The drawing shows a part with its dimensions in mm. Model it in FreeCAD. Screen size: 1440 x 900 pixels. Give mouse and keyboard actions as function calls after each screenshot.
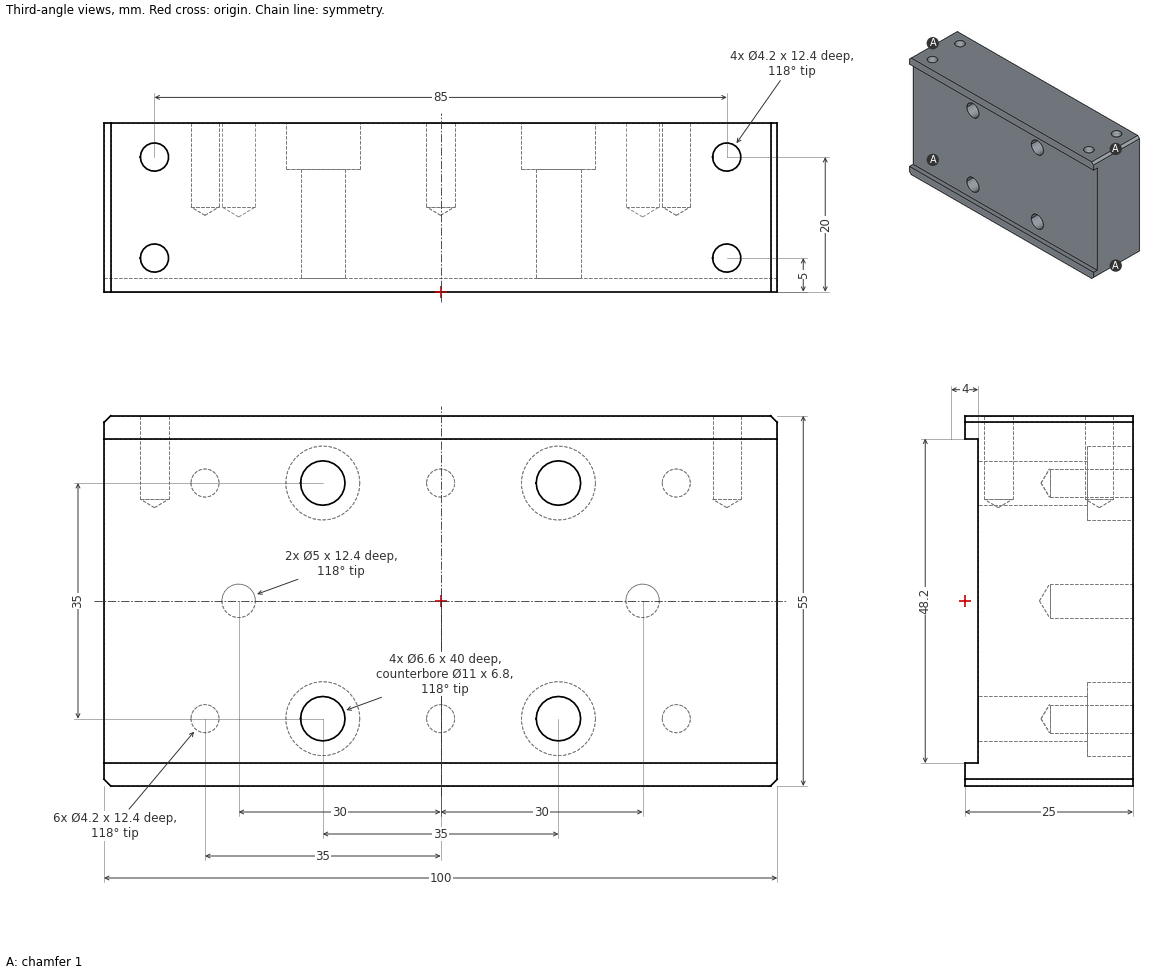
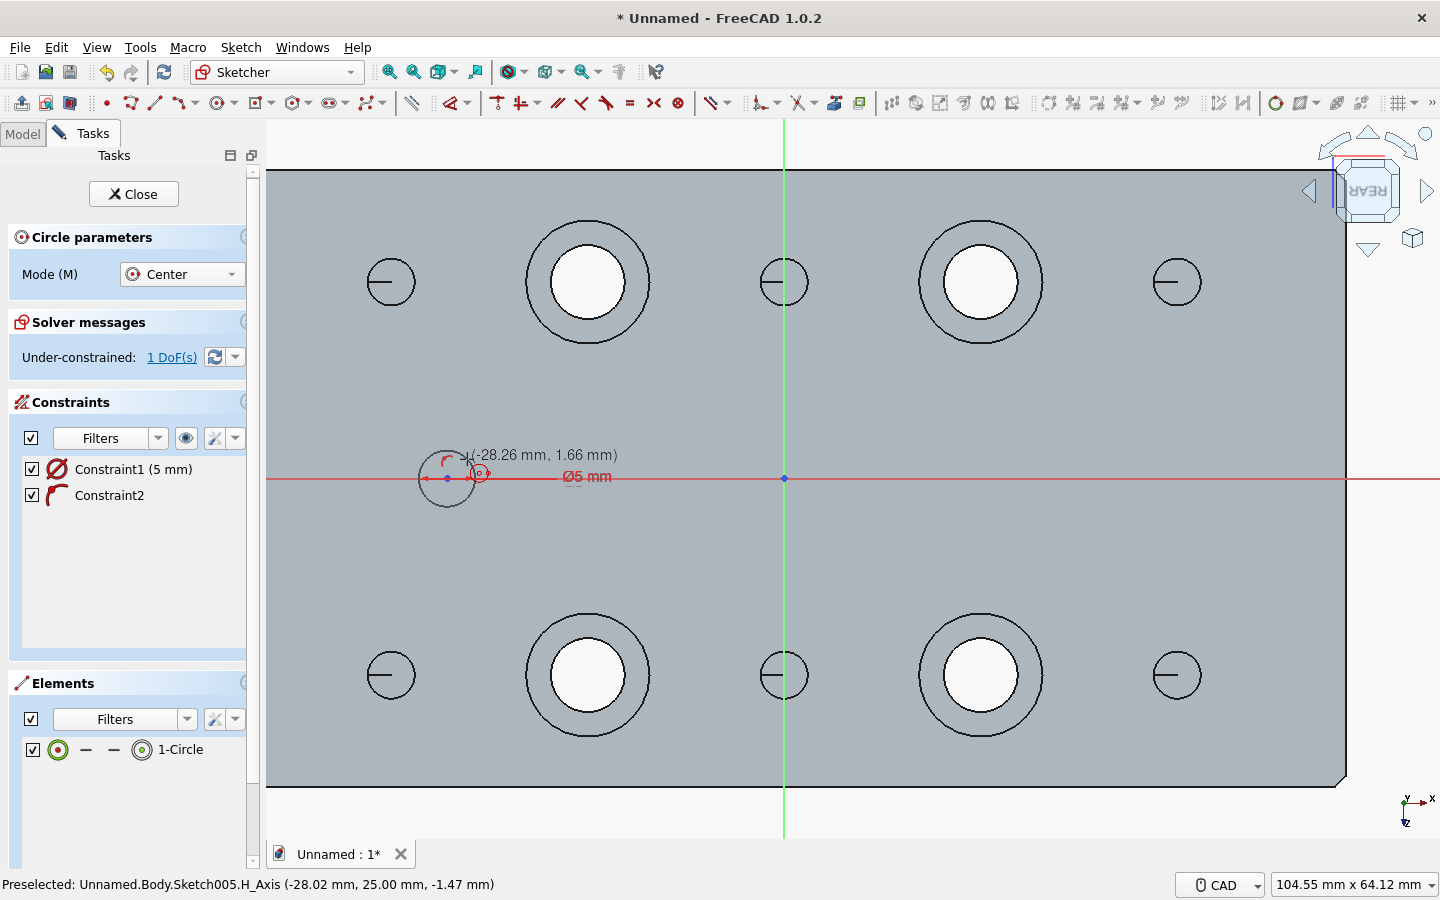
click(1121, 479)
move(1141, 459)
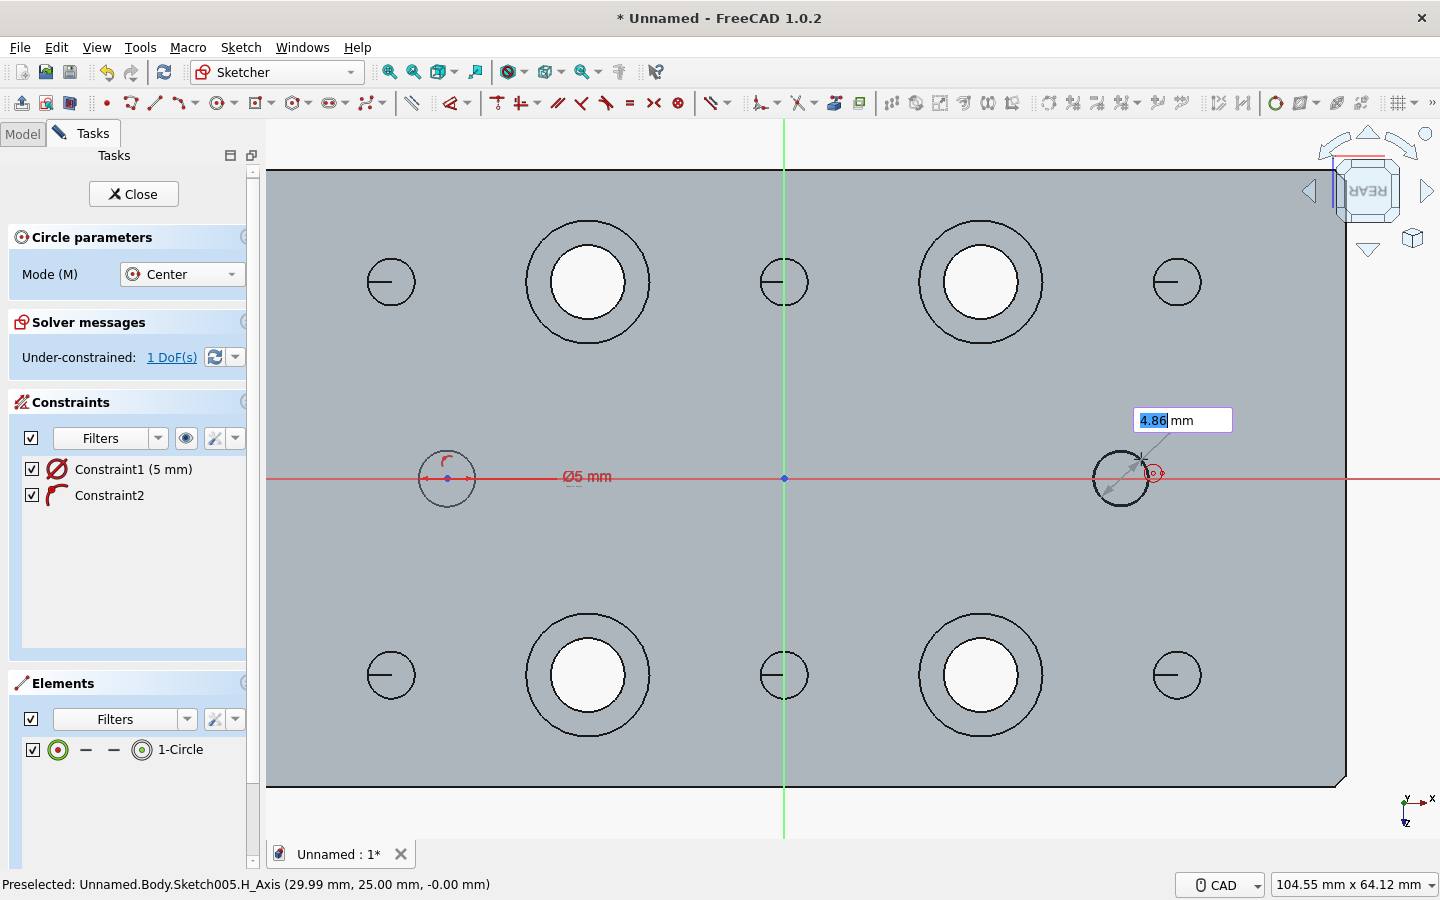
text(5)
key(Return)
key(Escape)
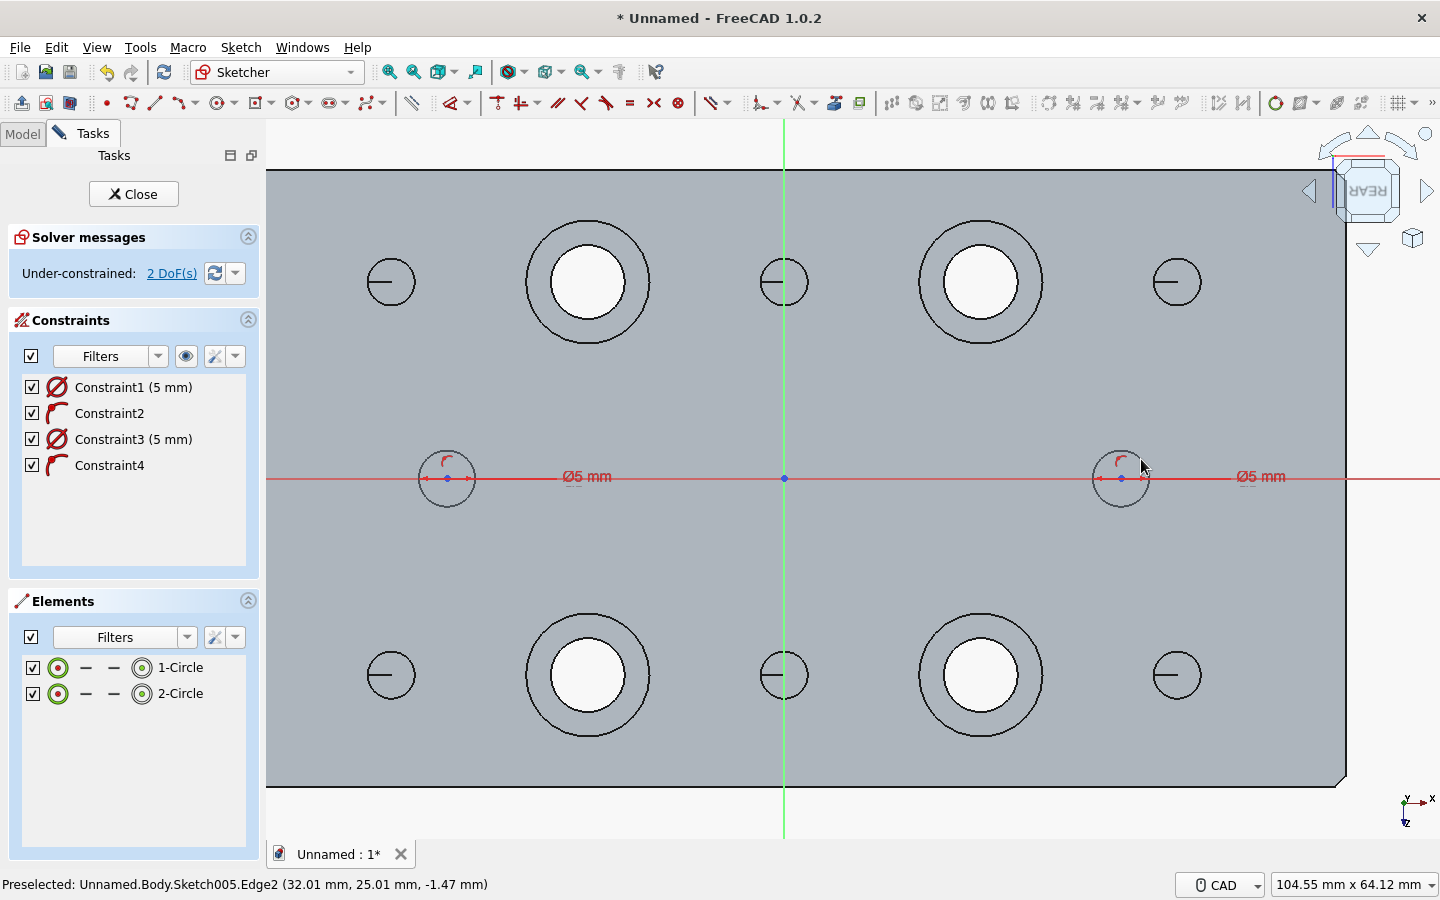
click(450, 104)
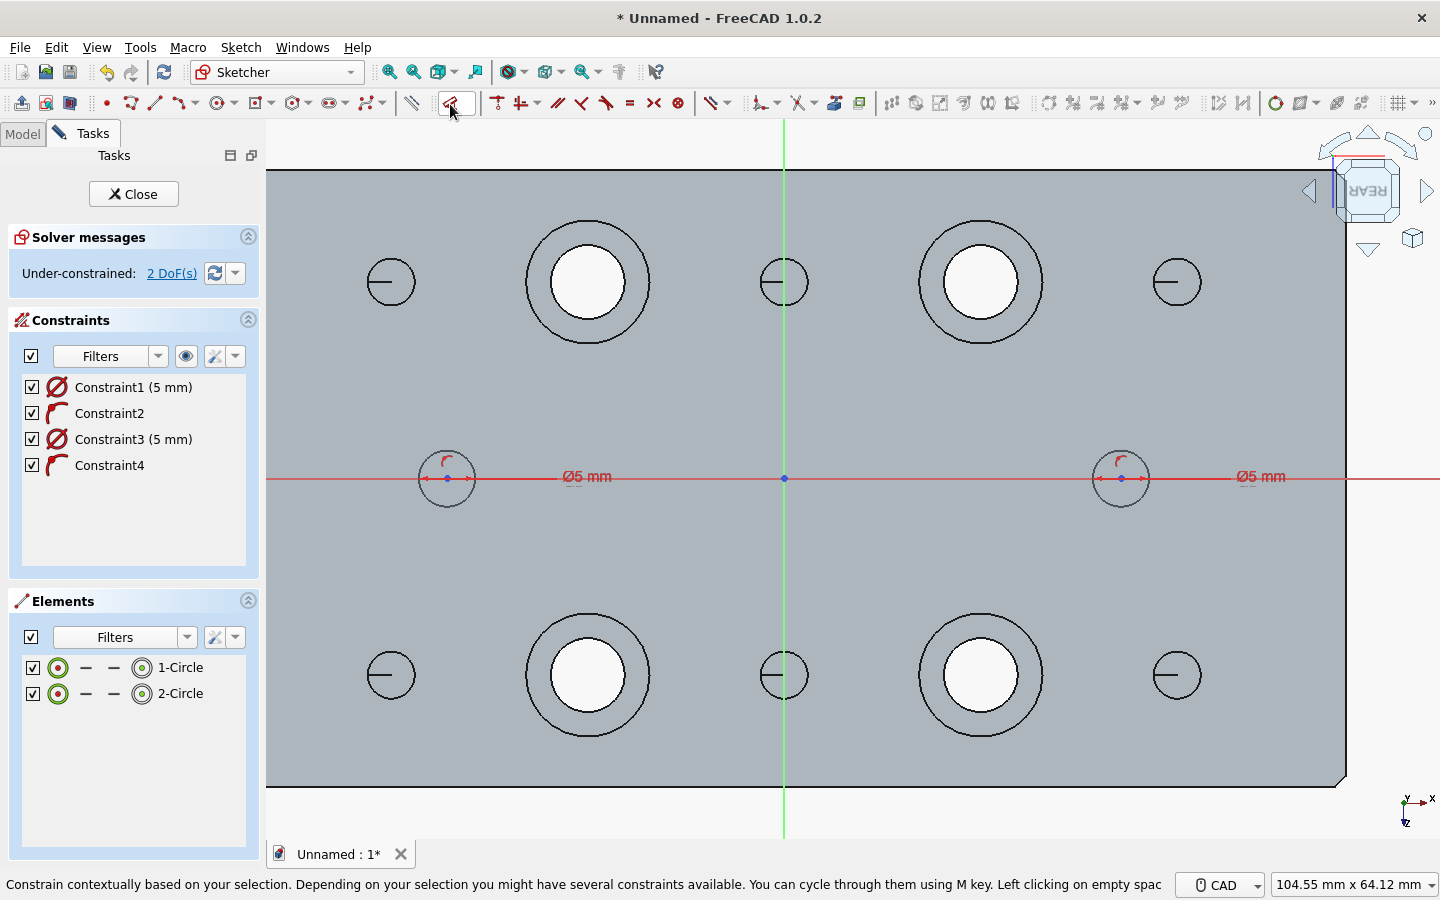
click(447, 479)
click(616, 513)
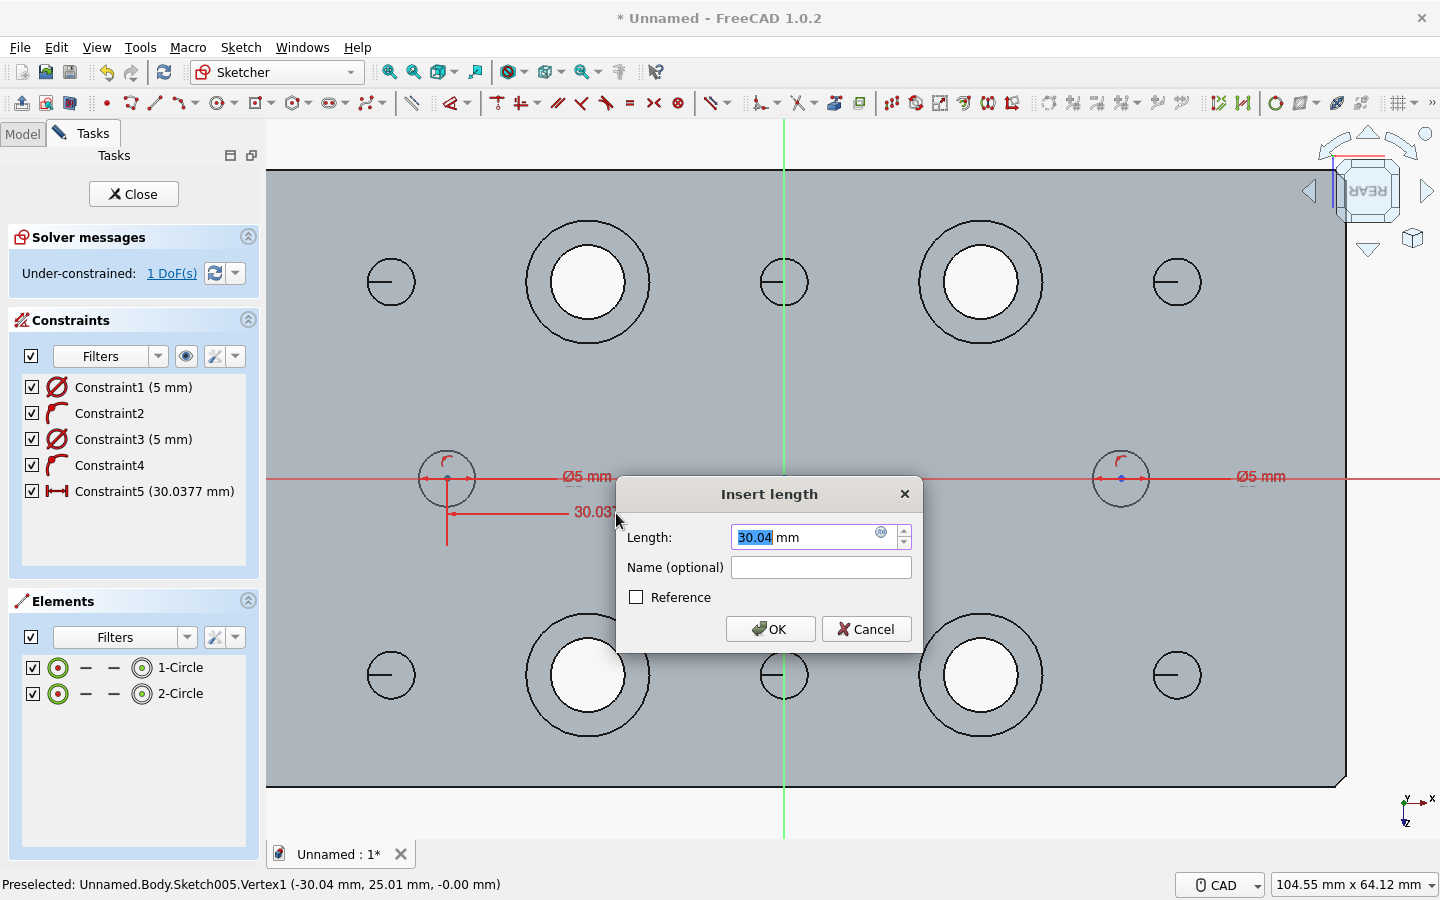
text(30)
key(Return)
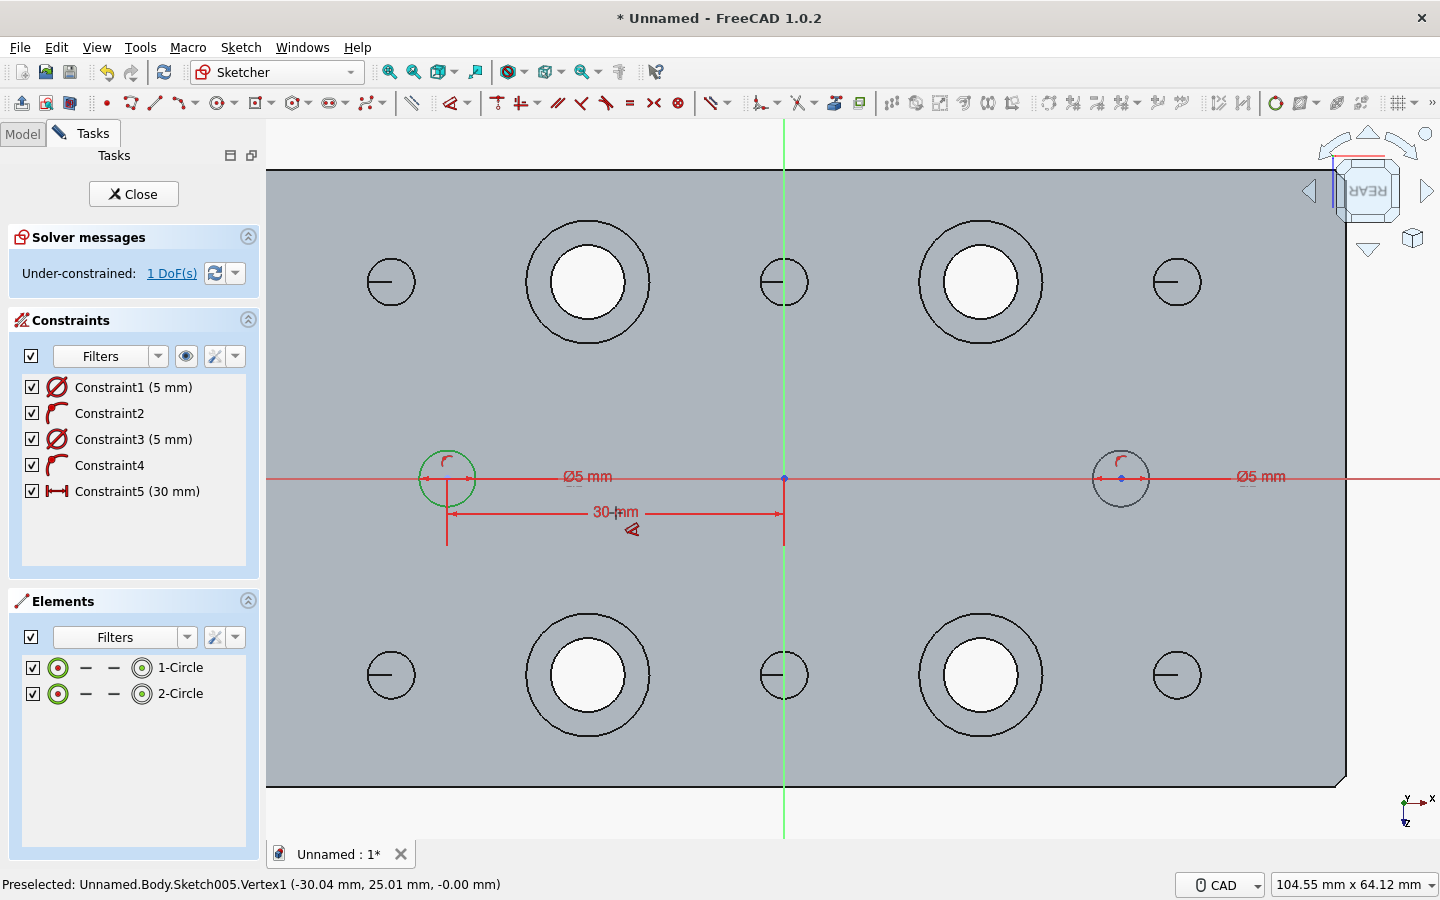
click(1121, 479)
click(953, 513)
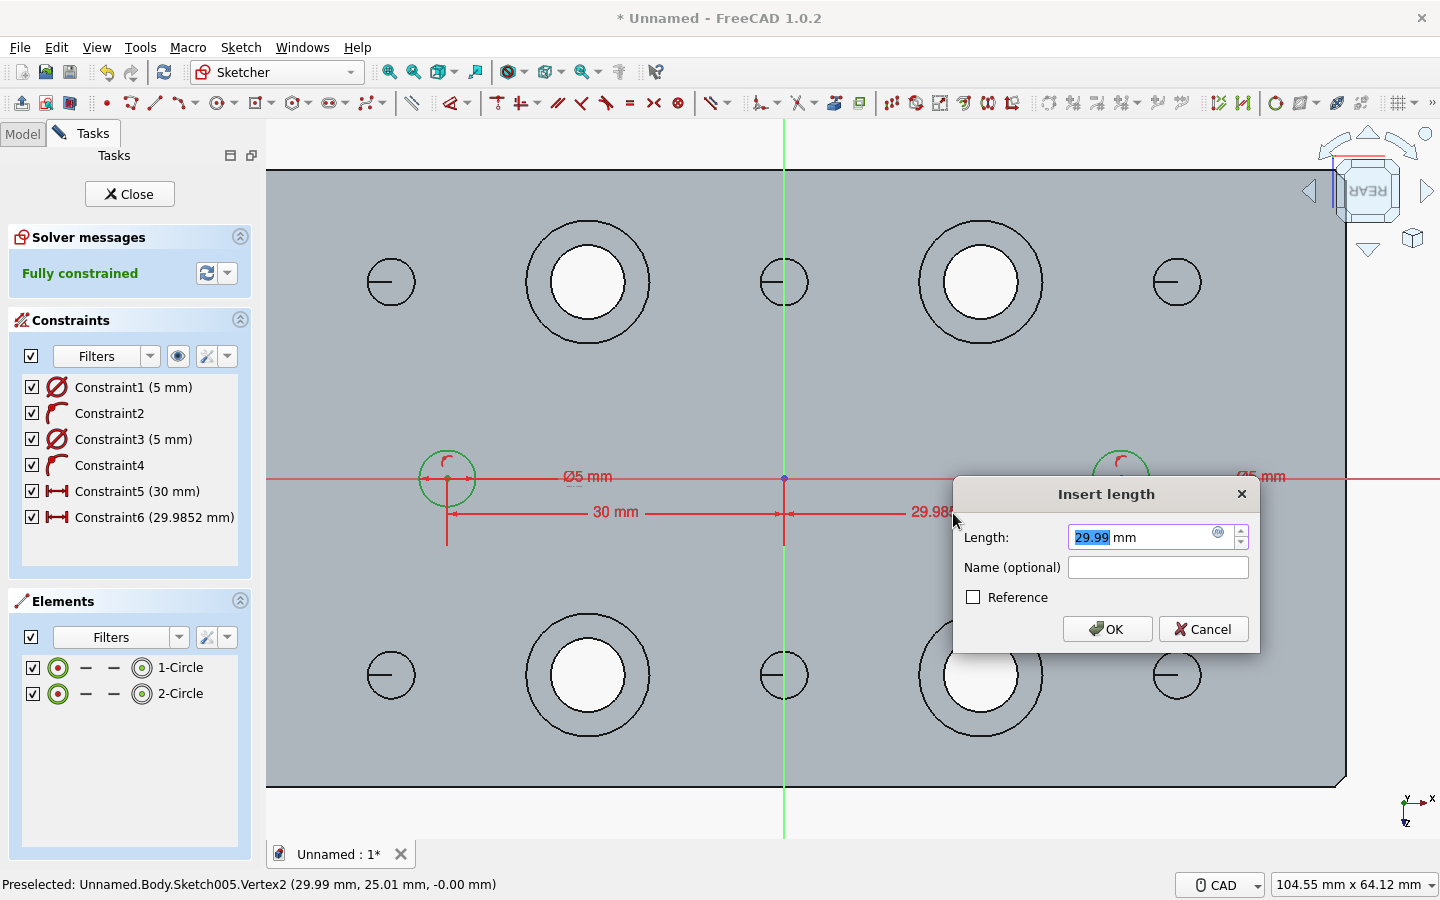
text(30)
key(Return)
key(Escape)